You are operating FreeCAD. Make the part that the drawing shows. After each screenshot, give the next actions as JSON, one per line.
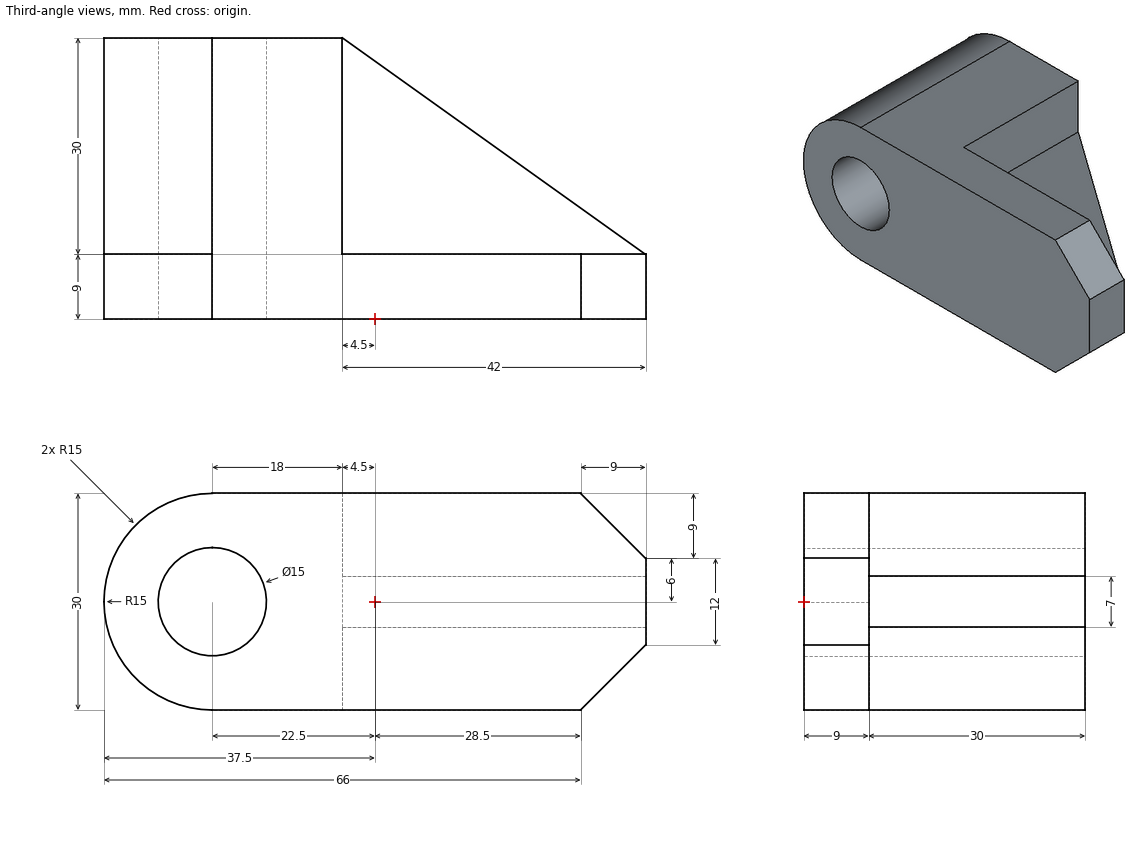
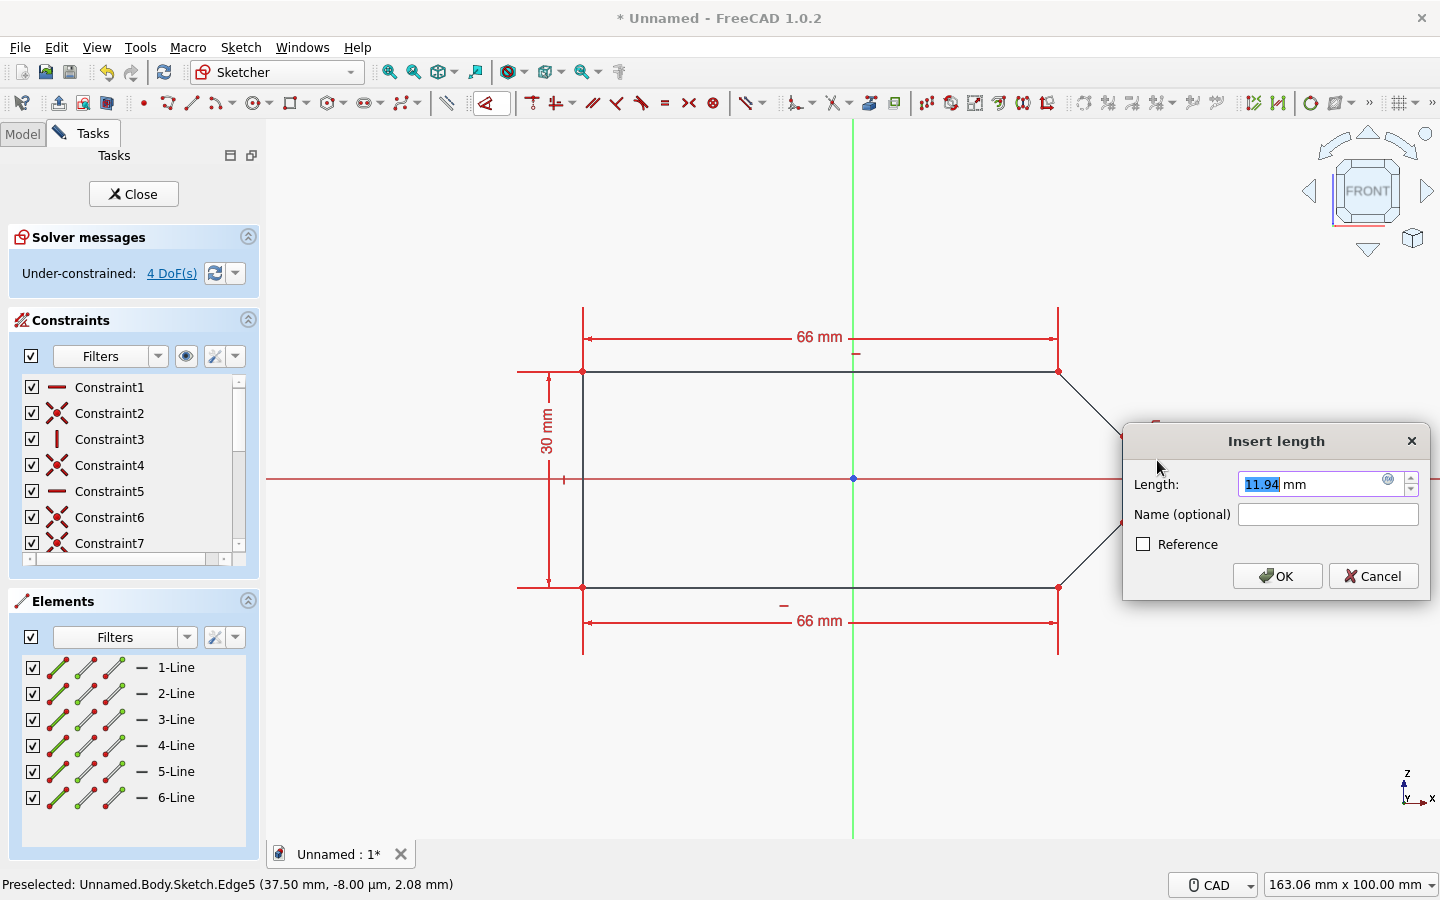
{"action": "type", "text": "12"}
{"action": "key", "text": "Return"}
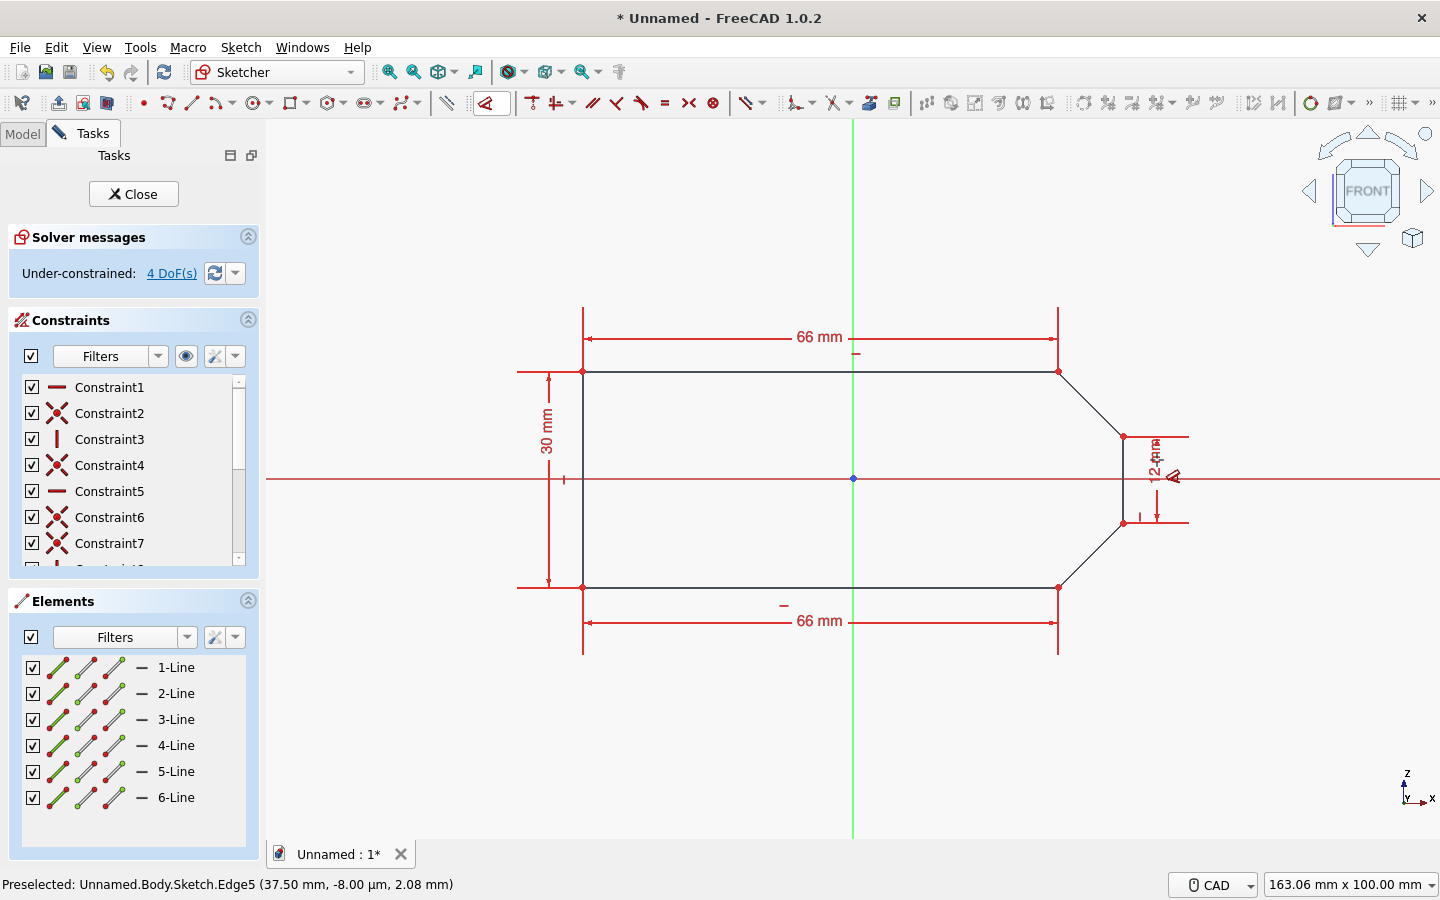
{"action": "left_click", "coordinate": [1123, 437]}
{"action": "left_click", "coordinate": [819, 458]}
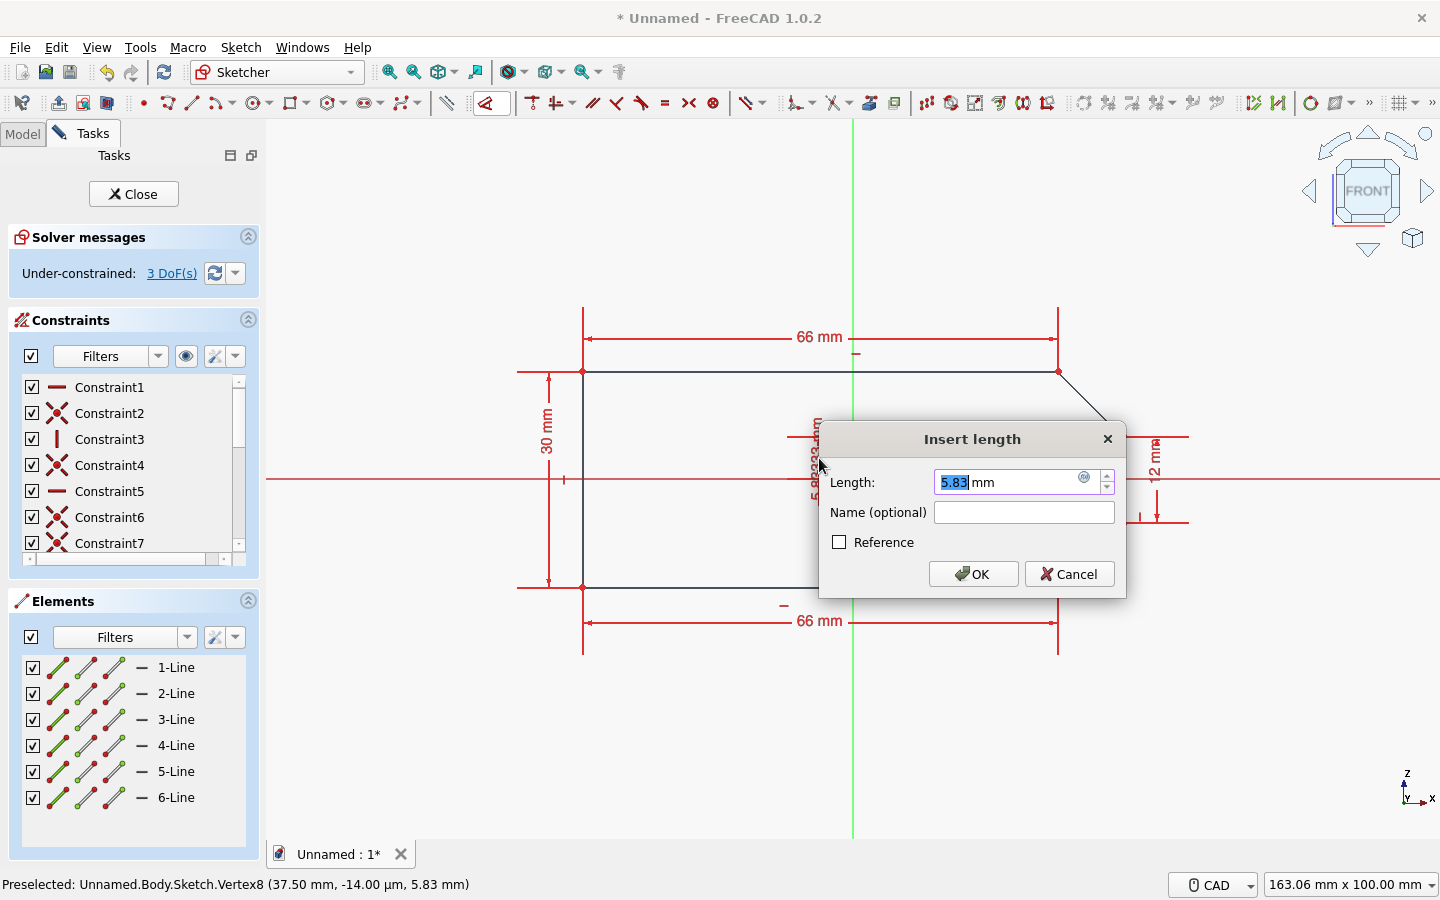
{"action": "type", "text": "6"}
{"action": "key", "text": "Return"}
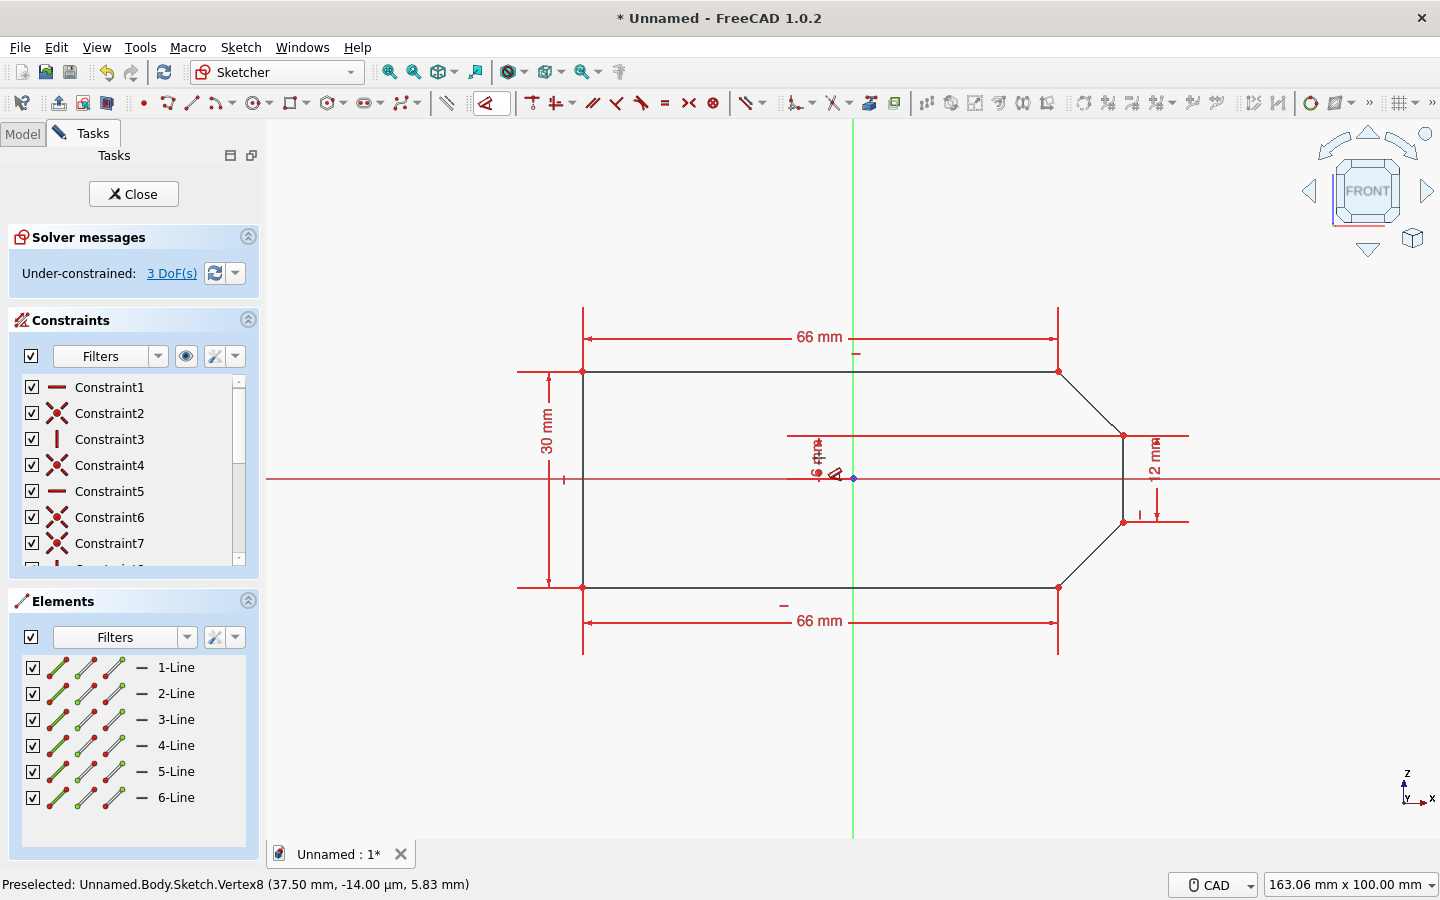
{"action": "left_click", "coordinate": [1077, 391]}
{"action": "left_click", "coordinate": [1090, 338]}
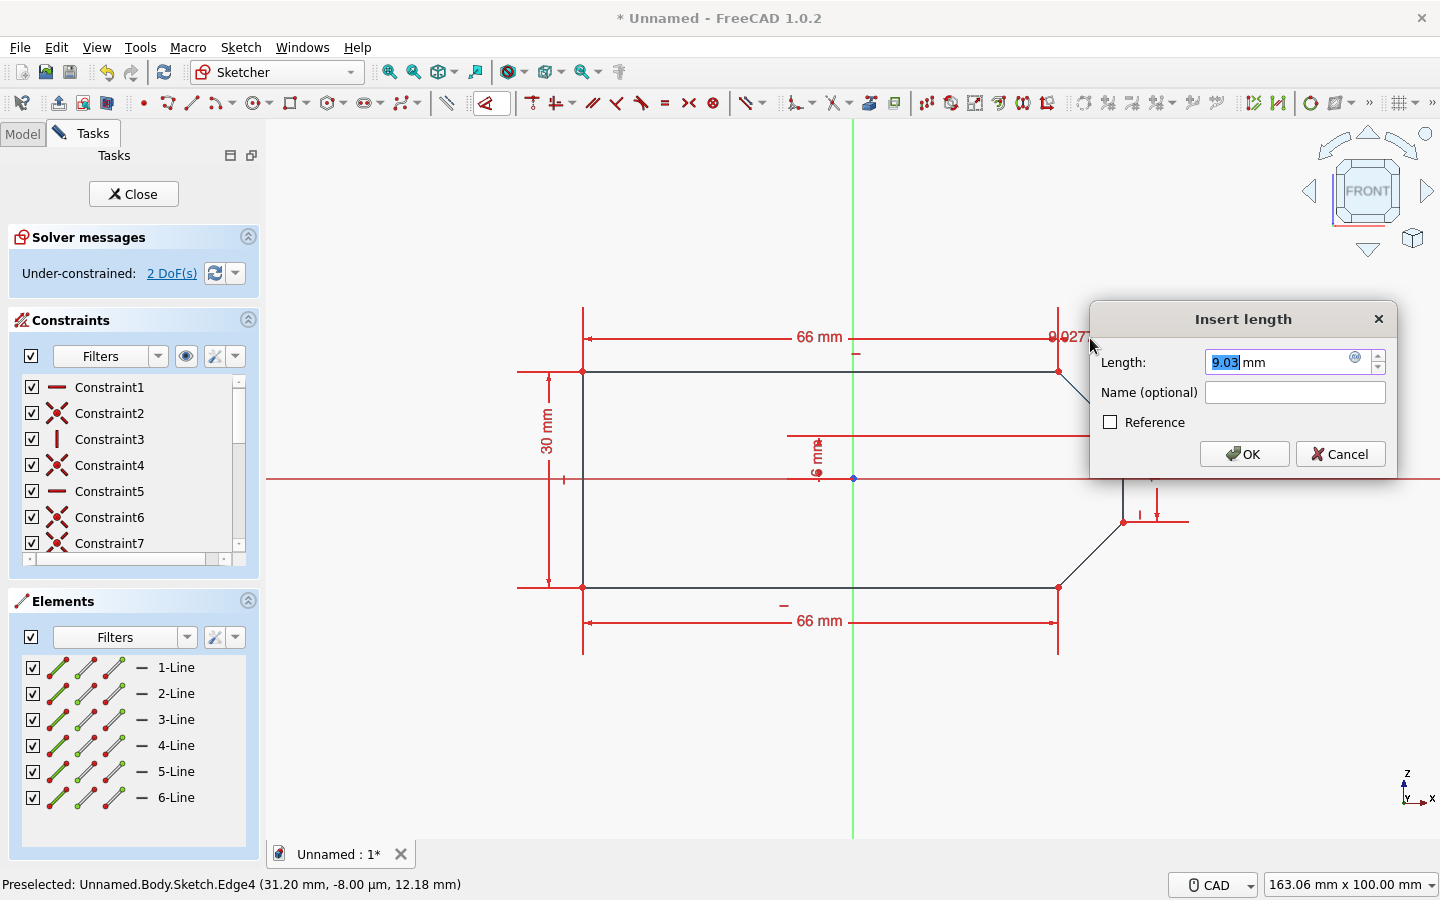
{"action": "type", "text": "9"}
{"action": "key", "text": "Return"}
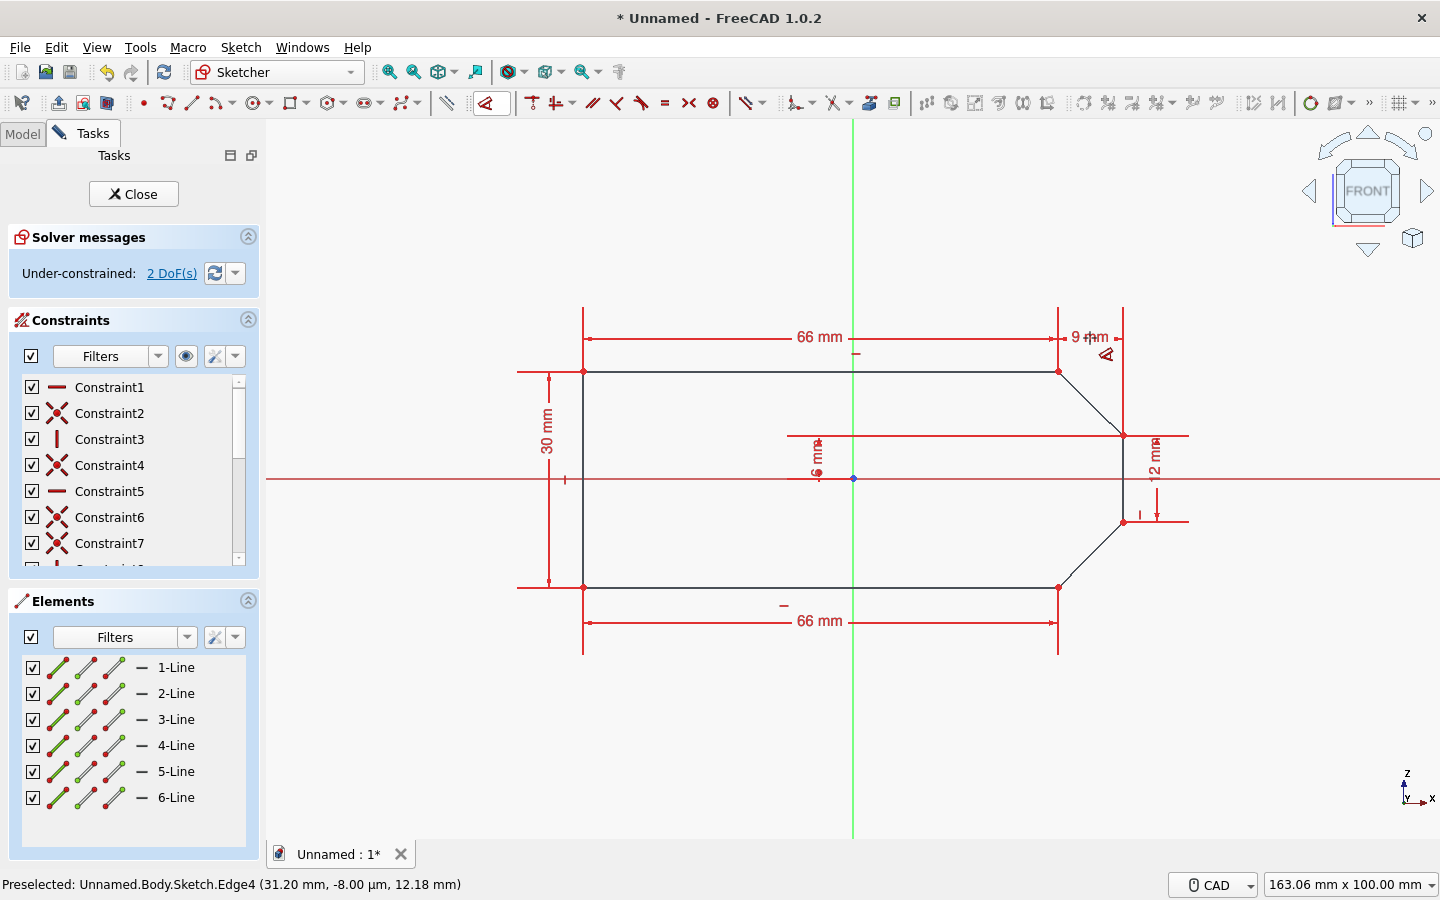
{"action": "left_click", "coordinate": [1078, 391]}
{"action": "left_click", "coordinate": [1157, 404]}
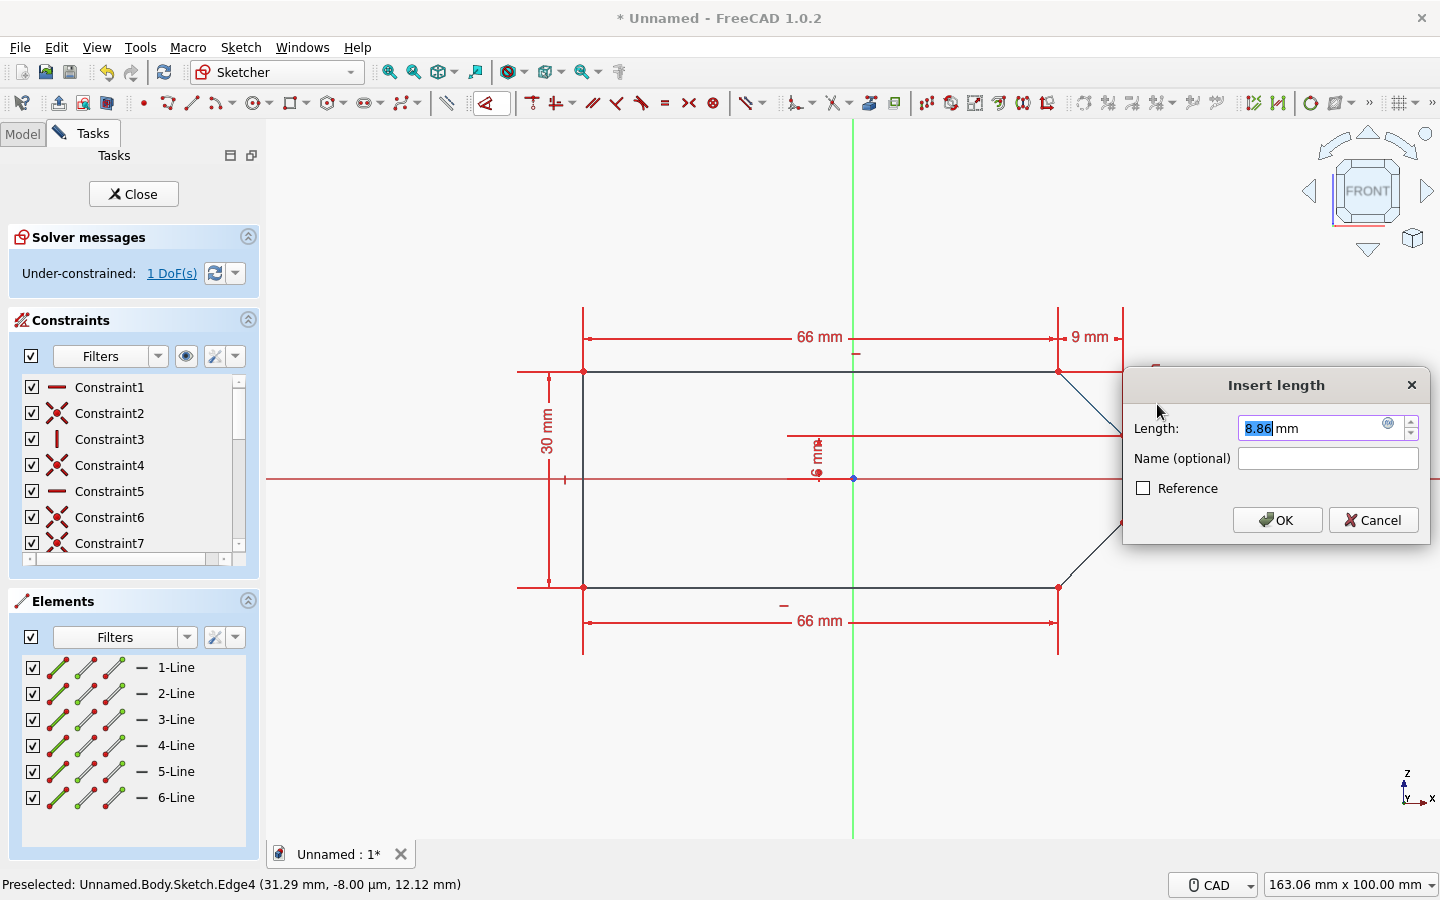
{"action": "type", "text": "9"}
{"action": "key", "text": "Return"}